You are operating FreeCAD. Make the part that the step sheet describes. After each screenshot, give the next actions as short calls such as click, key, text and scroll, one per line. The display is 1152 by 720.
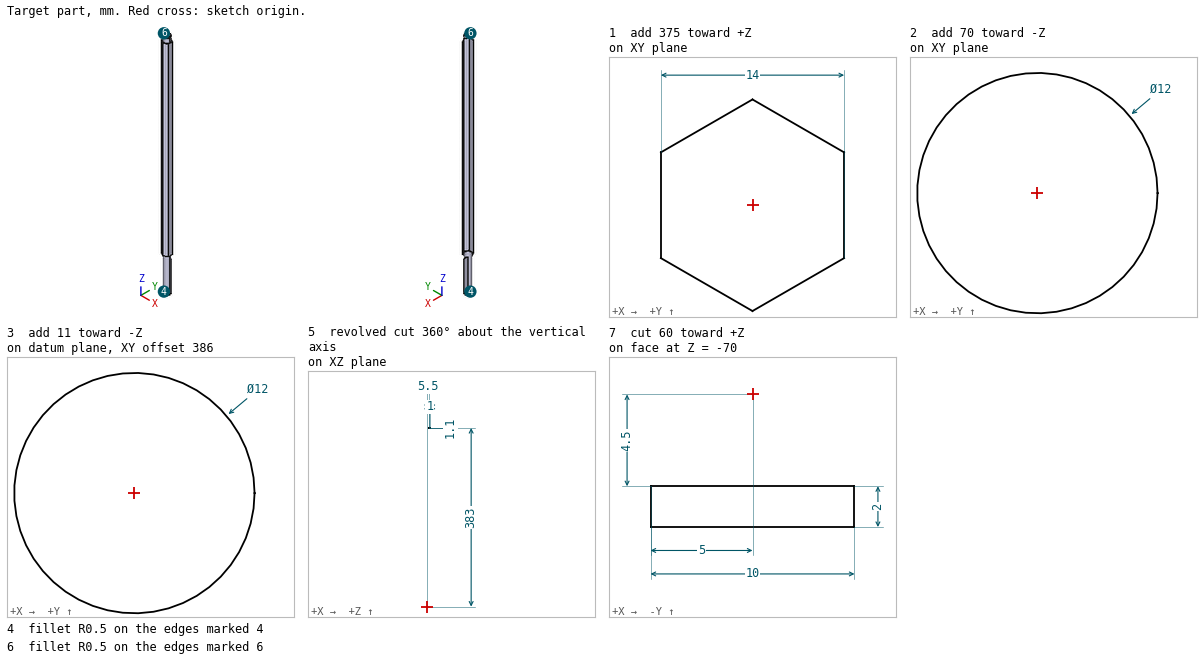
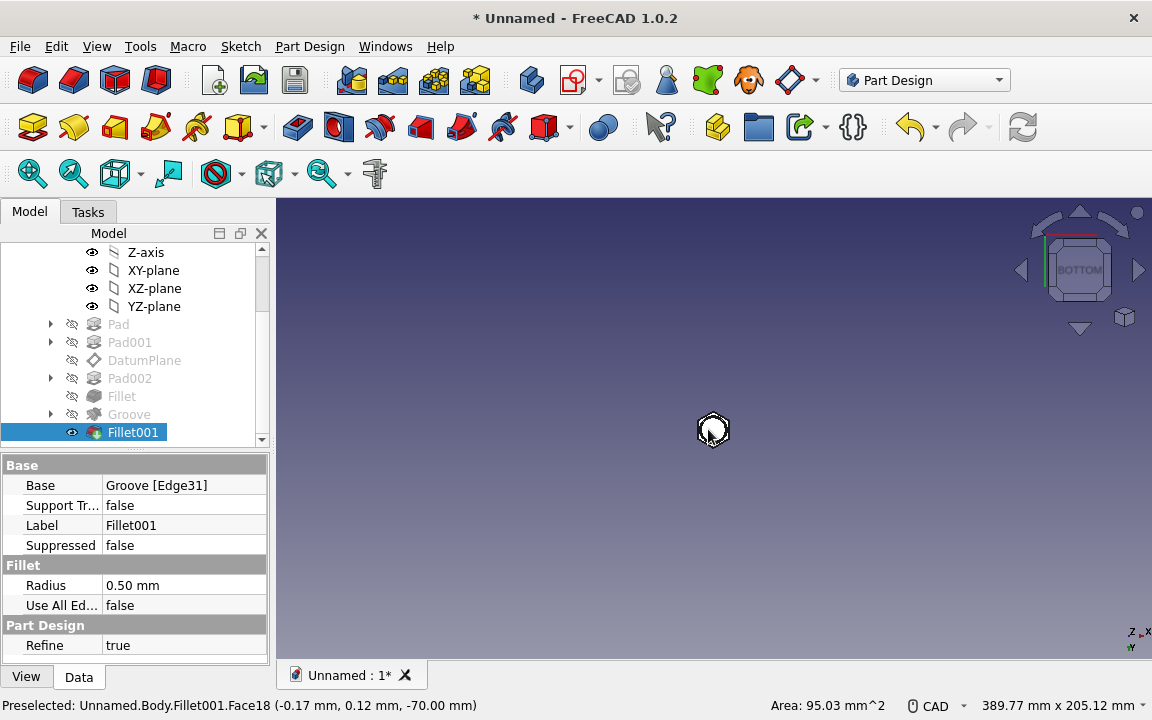
click(572, 80)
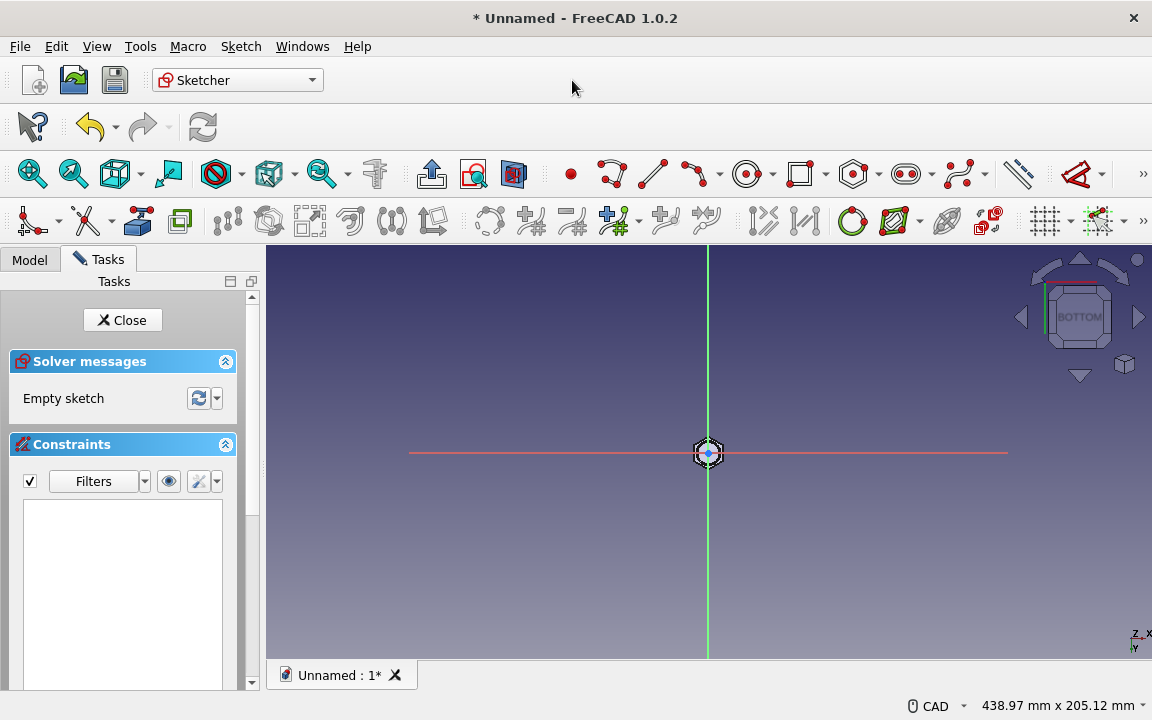
scroll(712, 460, up, 15)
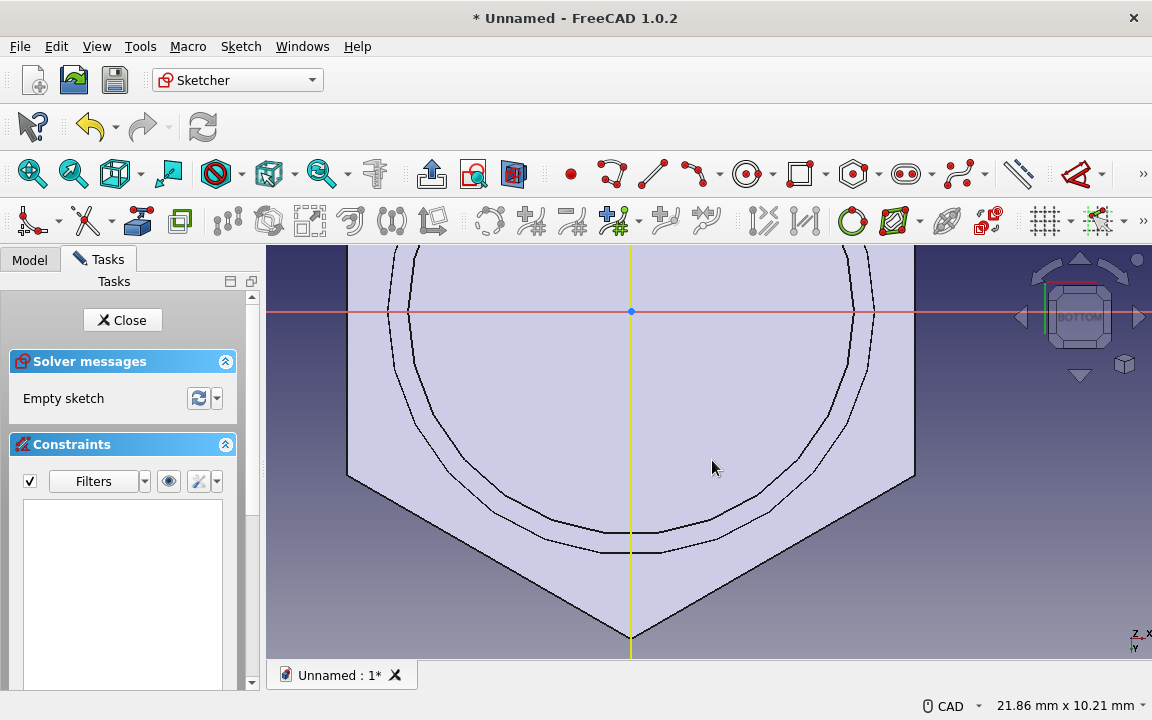
click(800, 174)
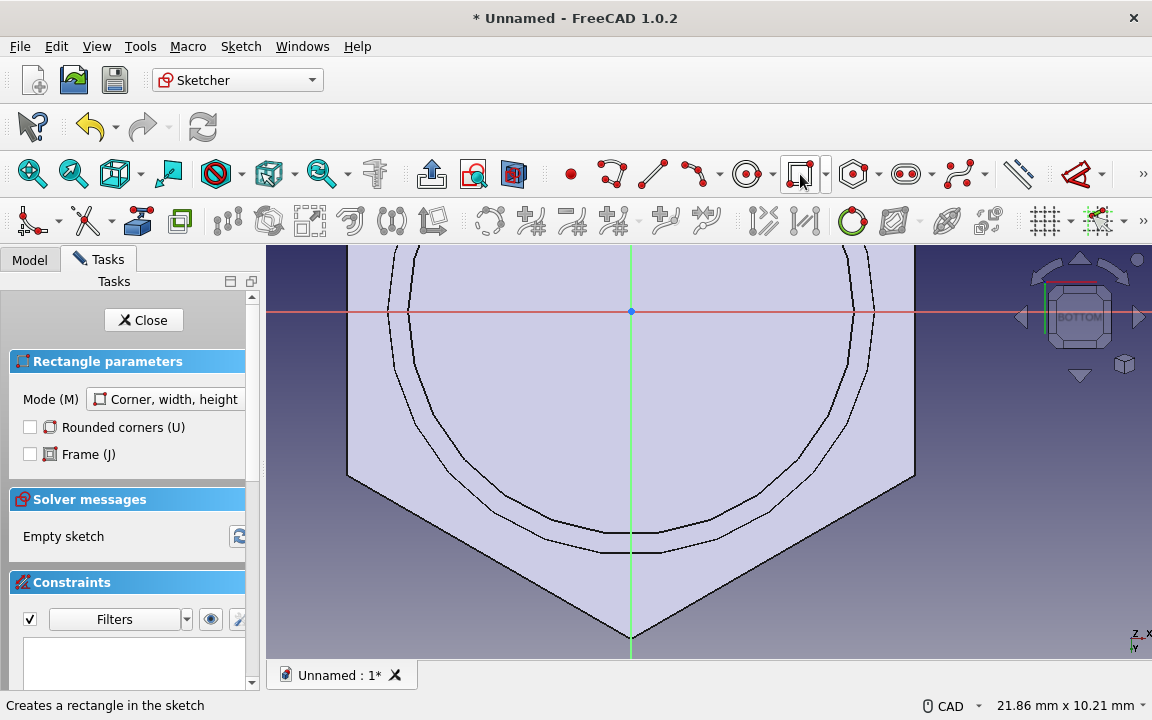
click(428, 494)
move(834, 575)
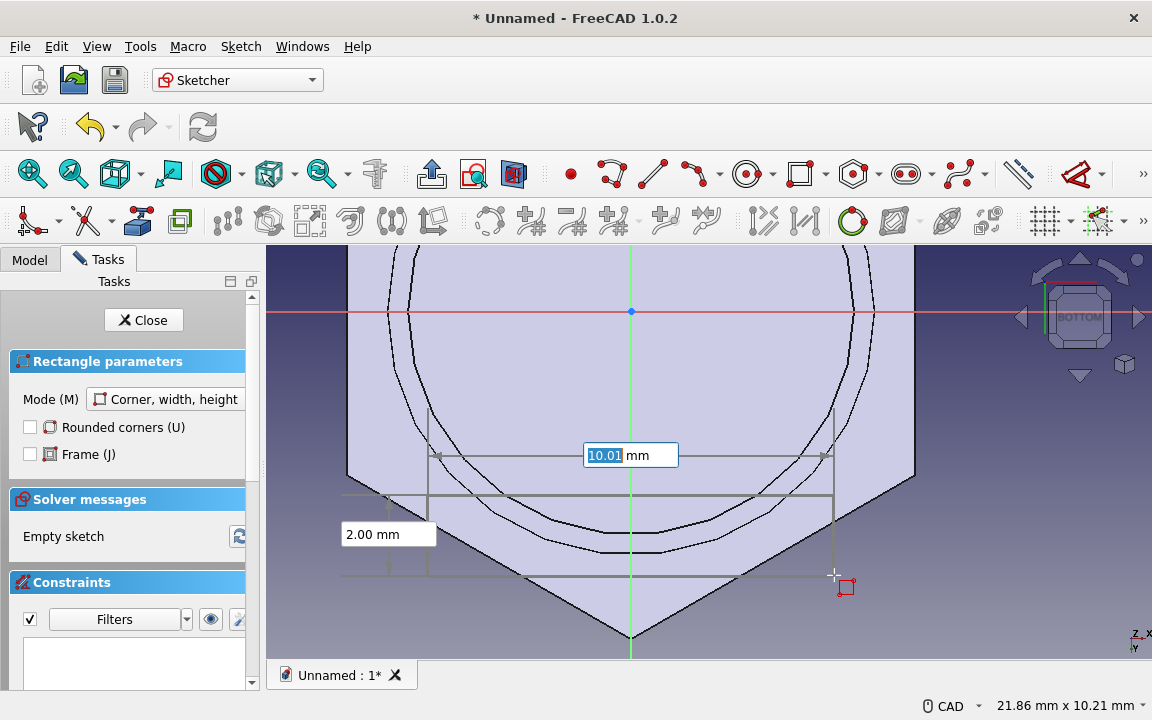
text(10)
key(Tab)
text(2)
key(Return)
key(Escape)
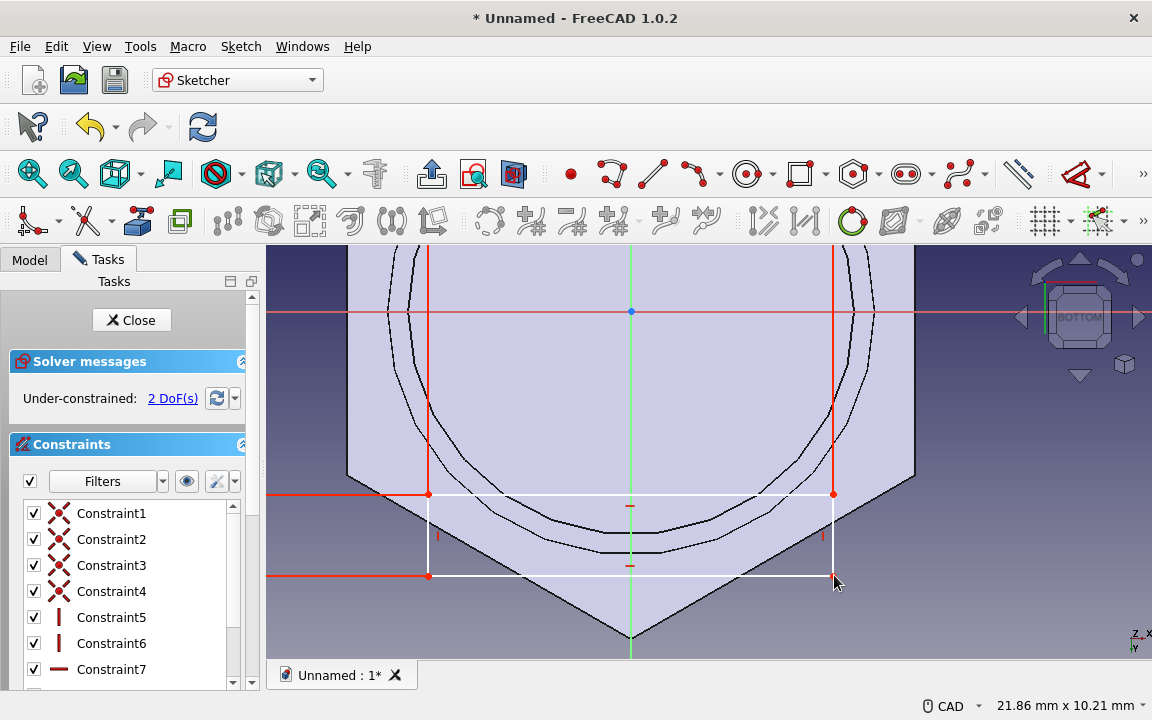
click(1076, 174)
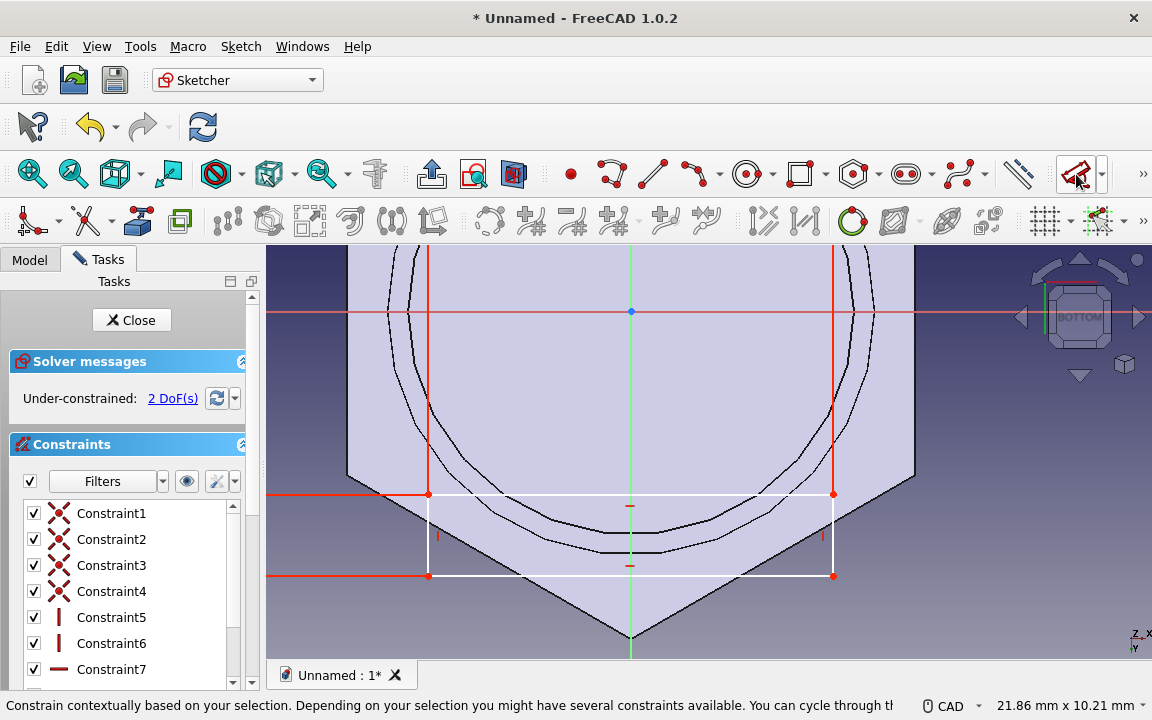
click(428, 495)
click(530, 278)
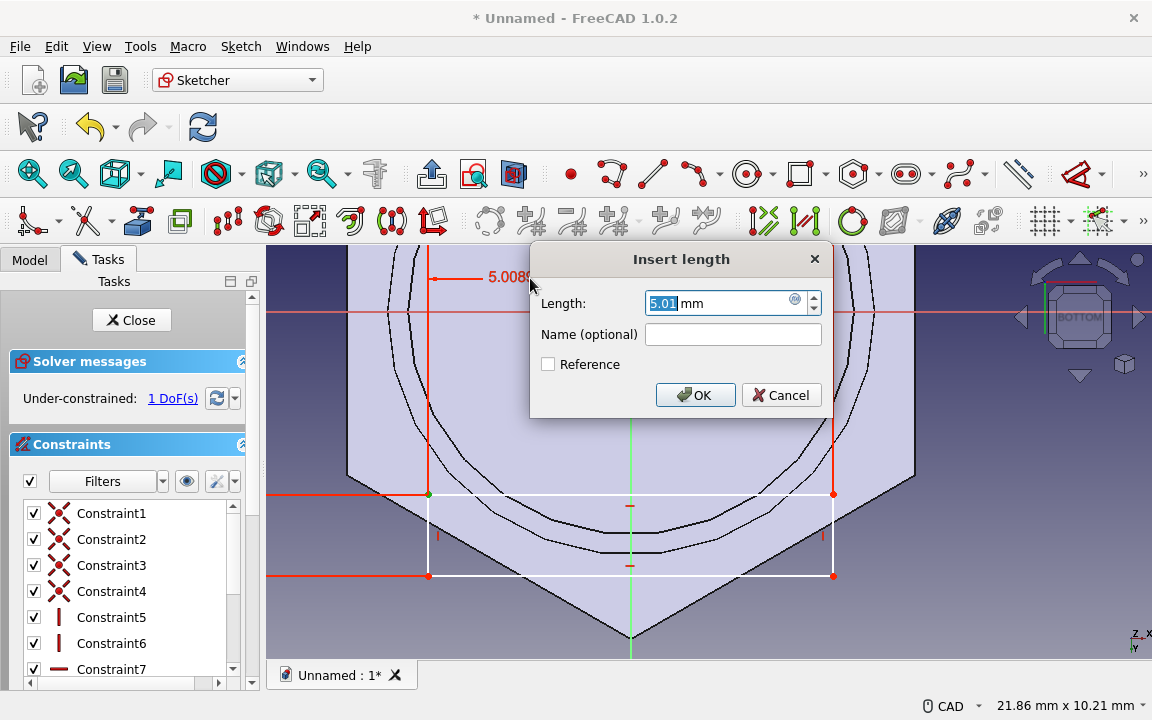
text(5)
key(Return)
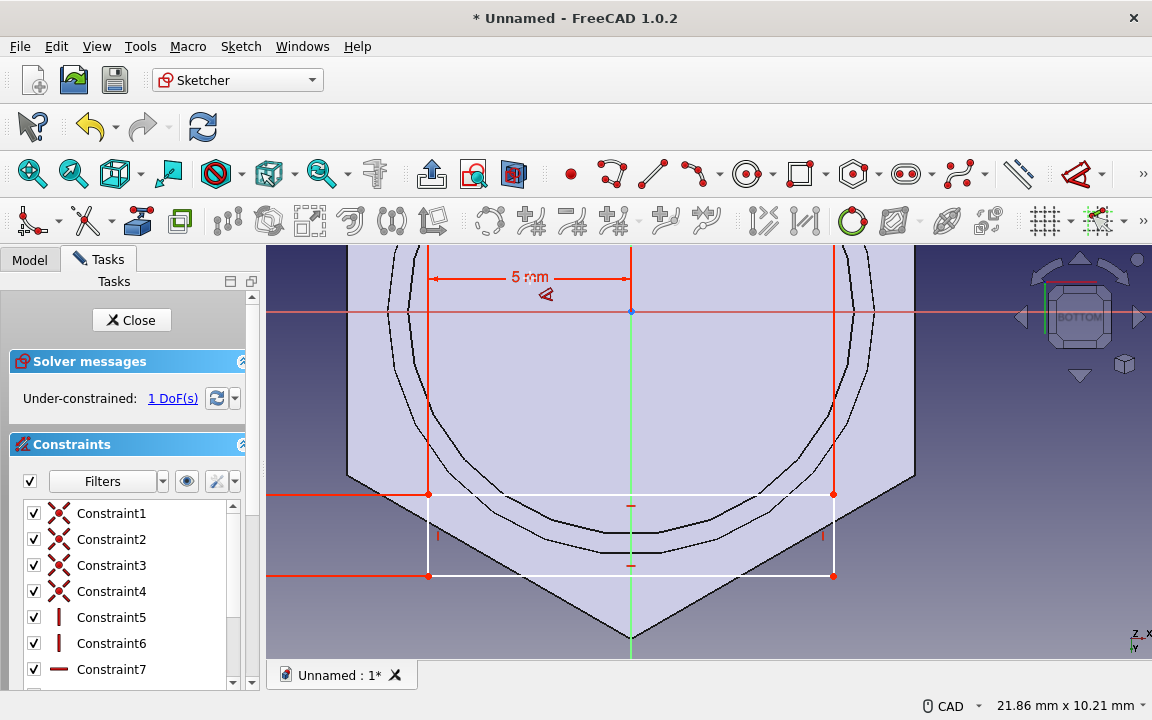
click(428, 495)
click(394, 403)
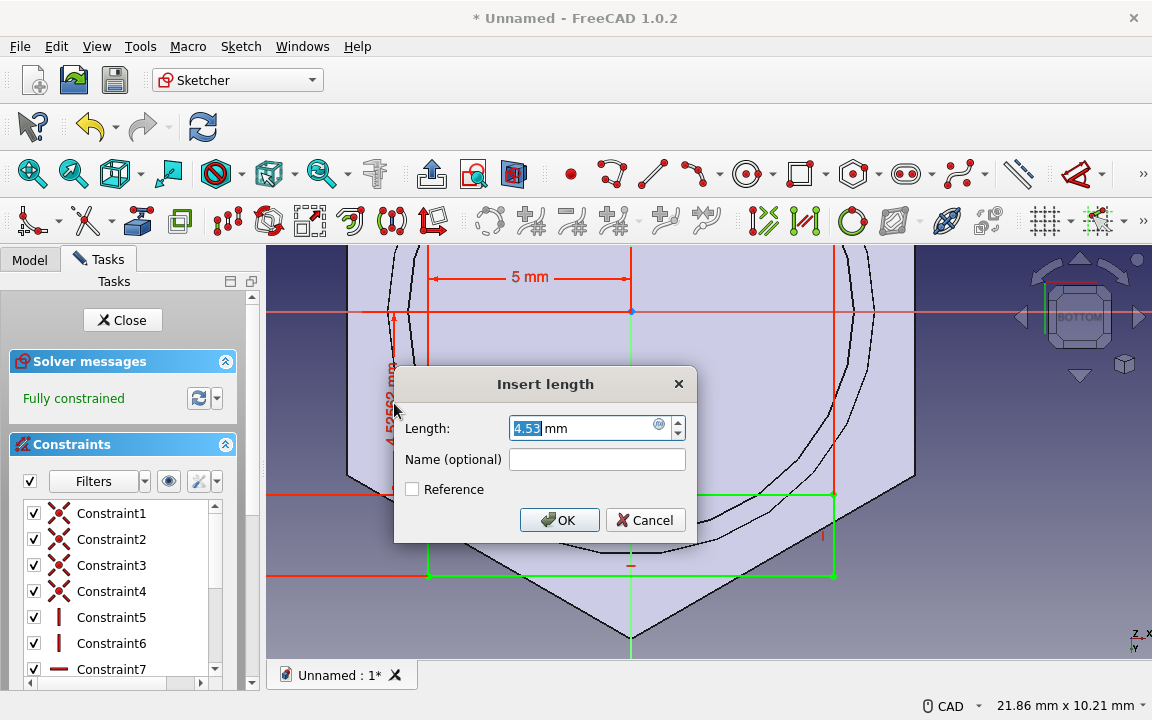
text(4.5)
key(Return)
key(Escape)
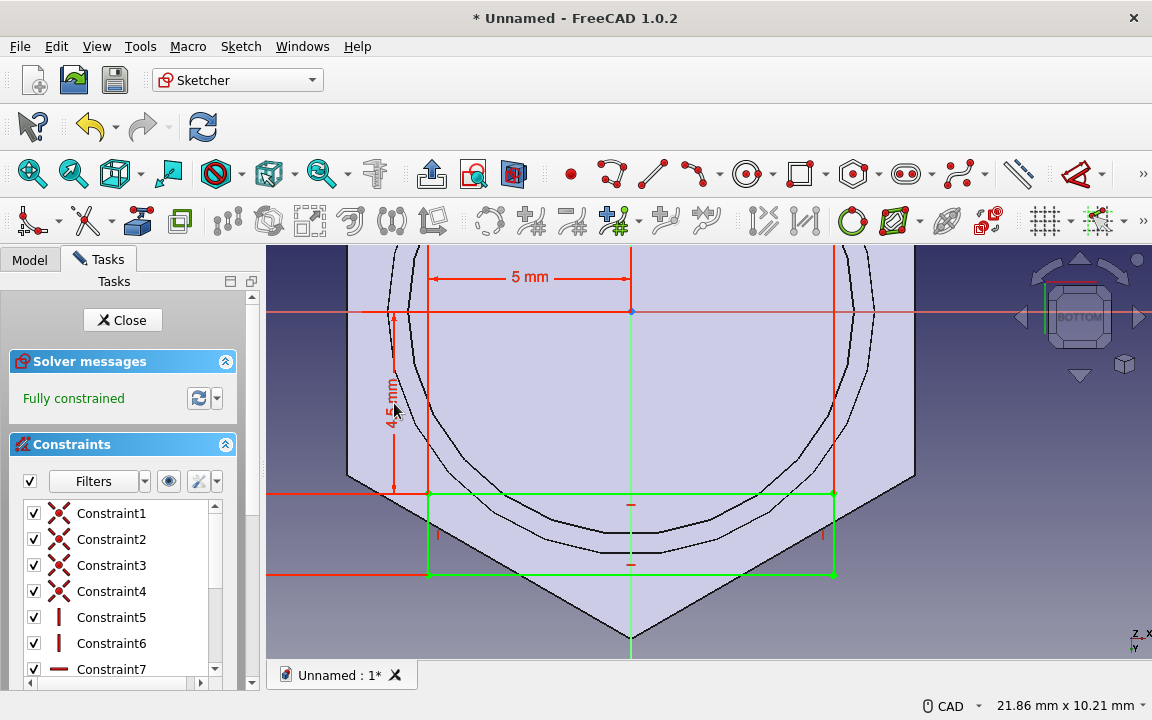
click(123, 320)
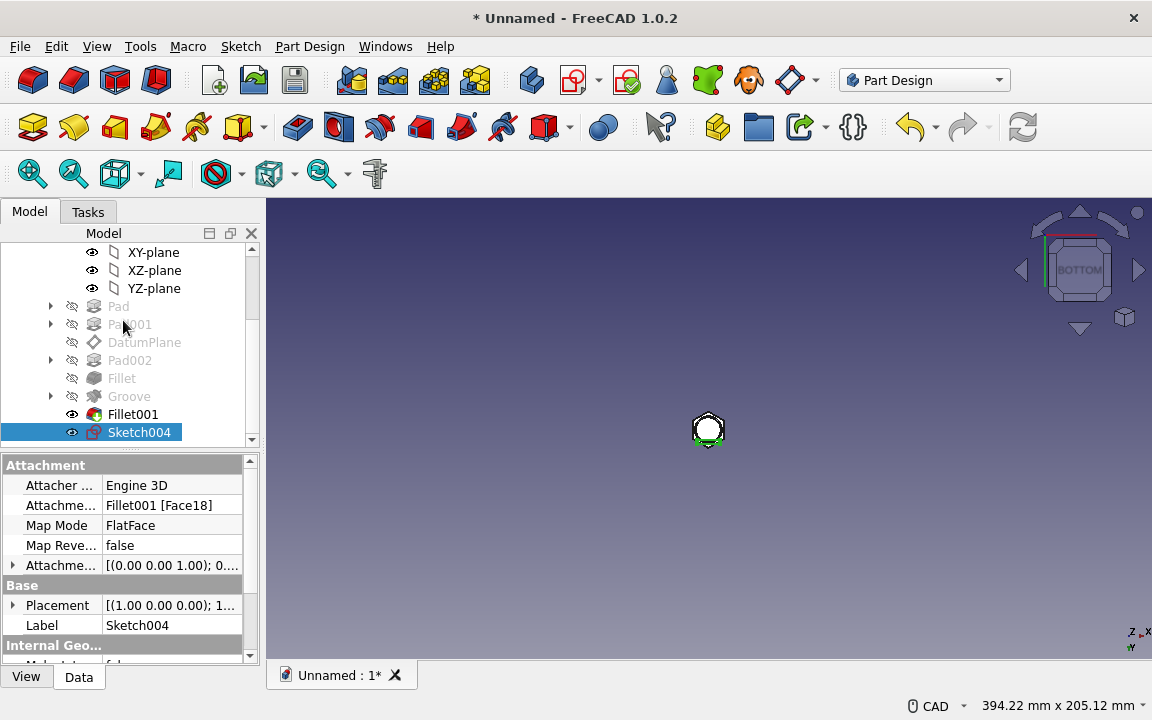
click(298, 128)